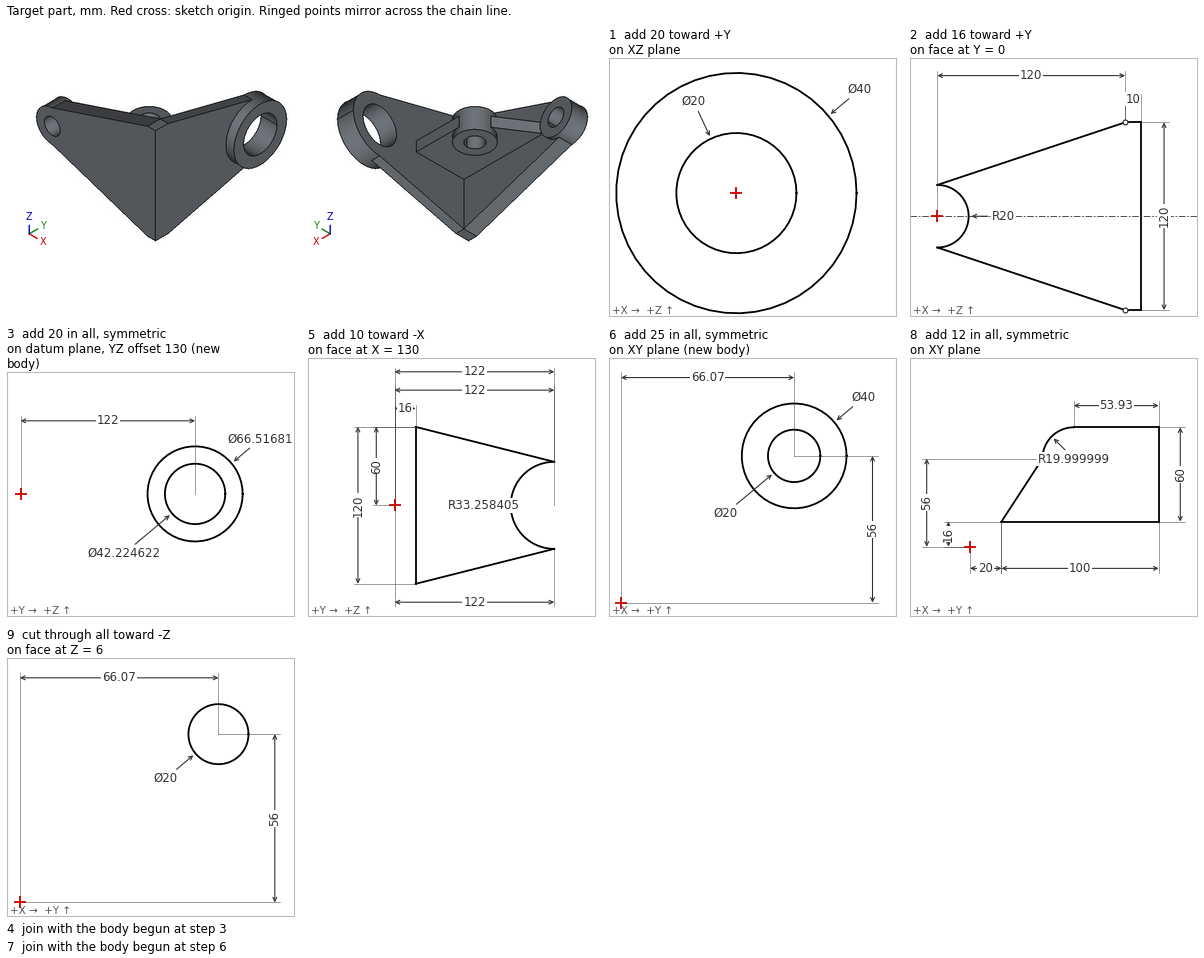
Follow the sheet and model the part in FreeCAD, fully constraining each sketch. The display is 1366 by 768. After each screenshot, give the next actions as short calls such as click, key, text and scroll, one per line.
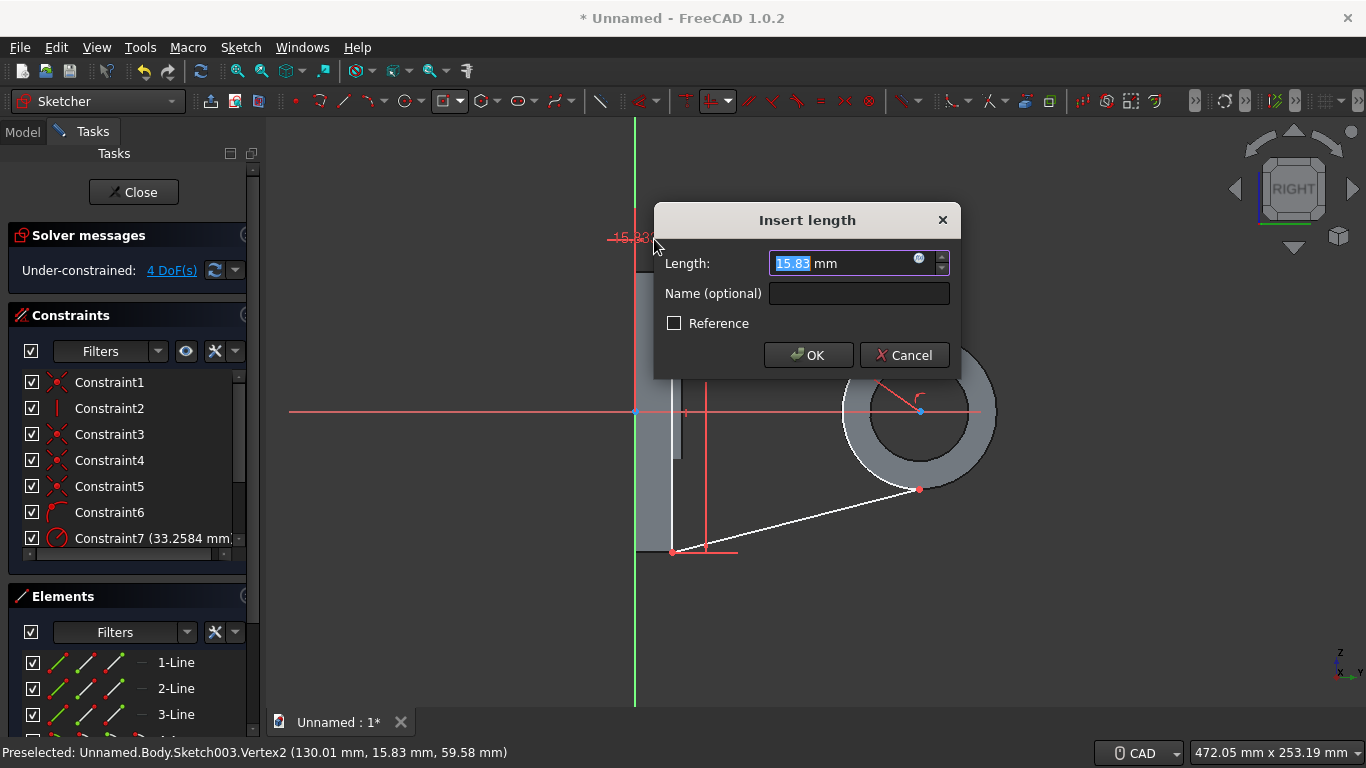
text(16)
key(Return)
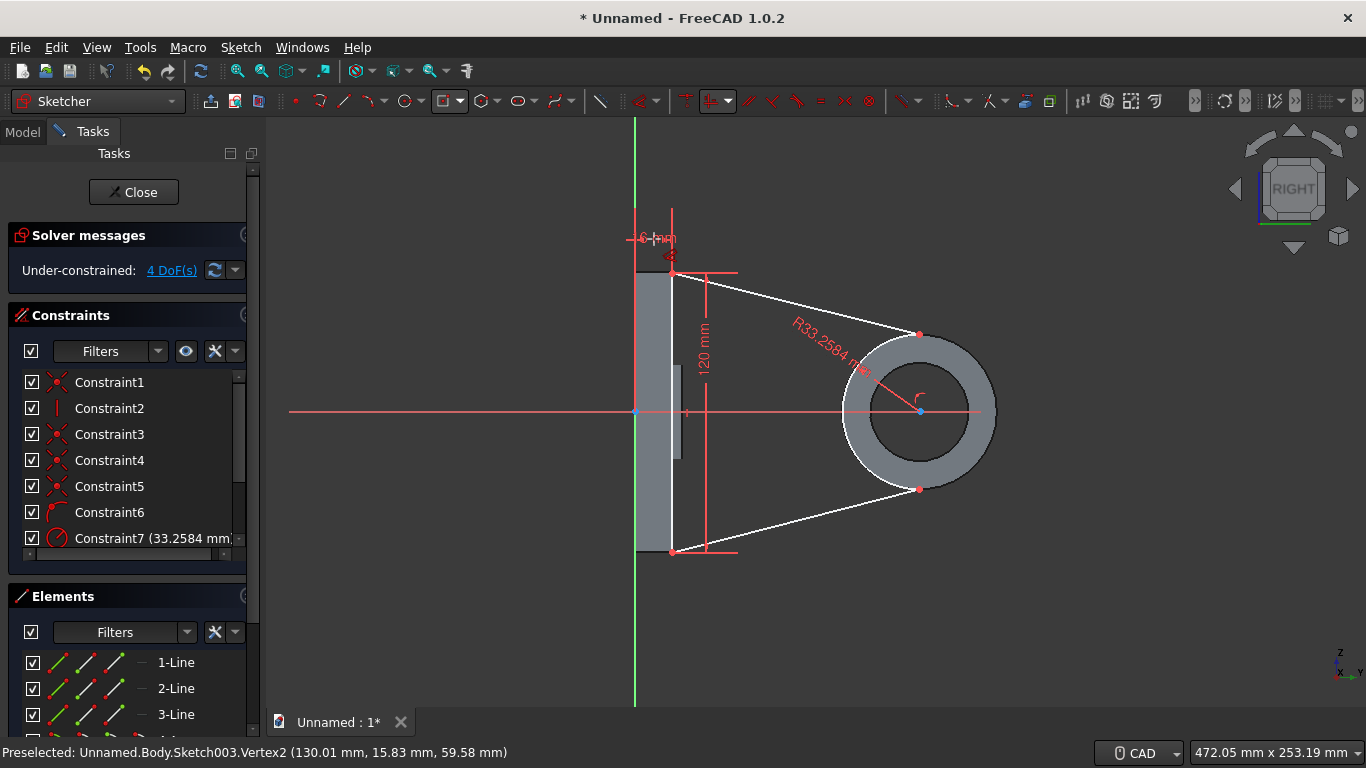
click(672, 273)
click(601, 343)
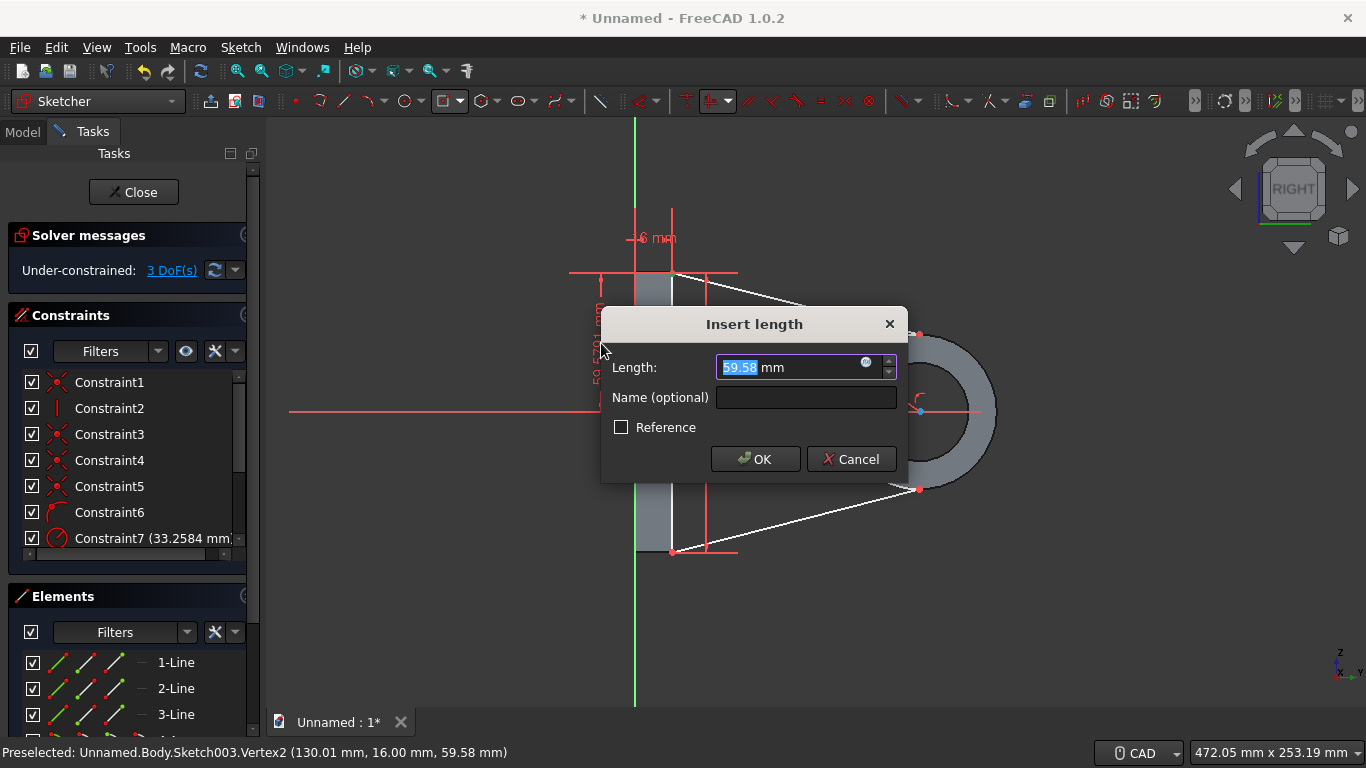
text(60)
key(Return)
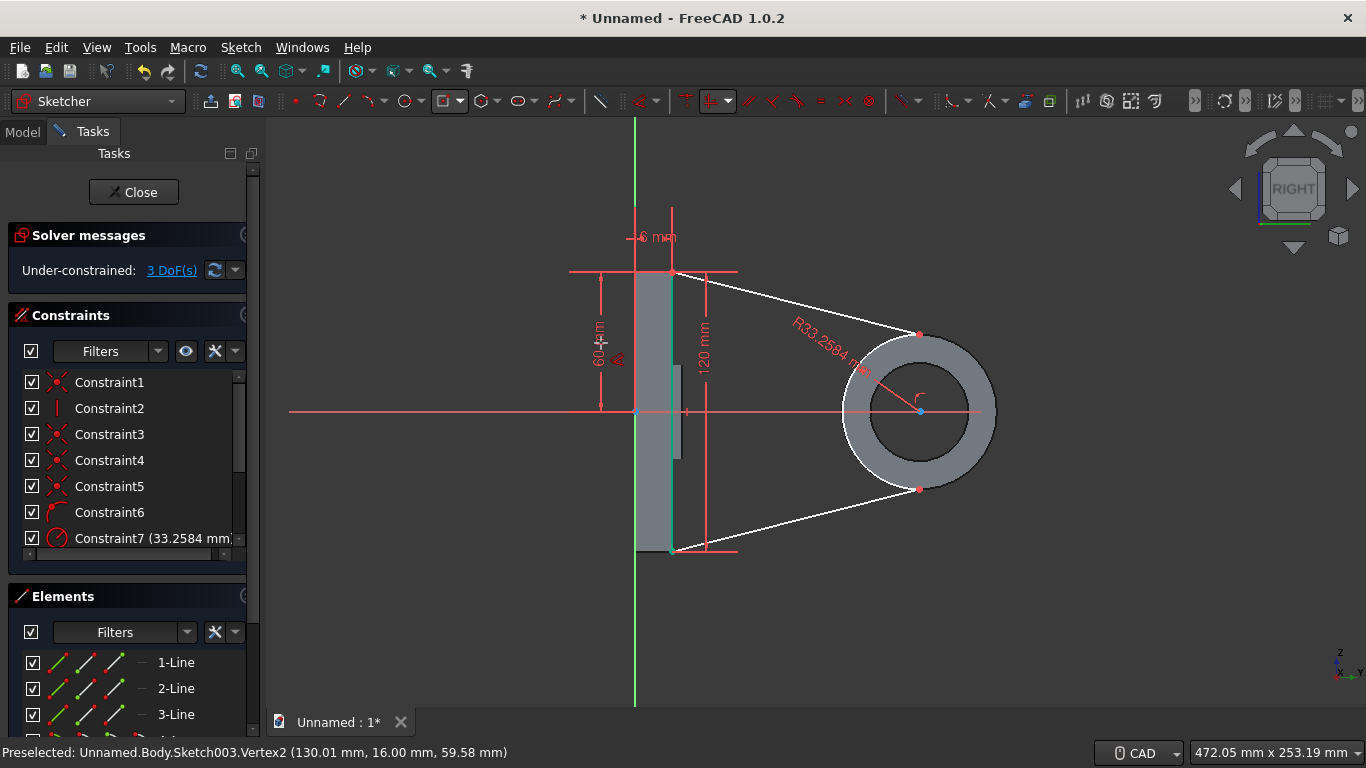
click(919, 335)
click(712, 301)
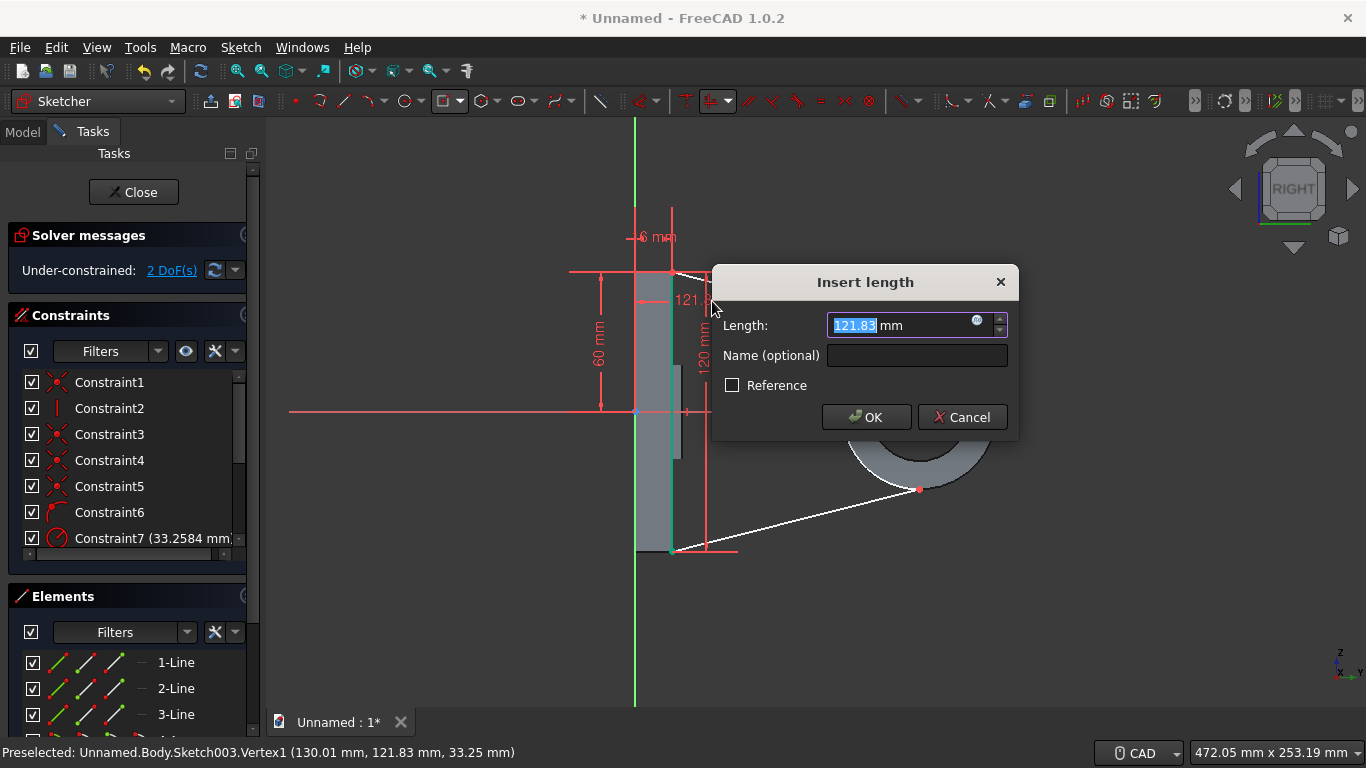
text(122)
key(Return)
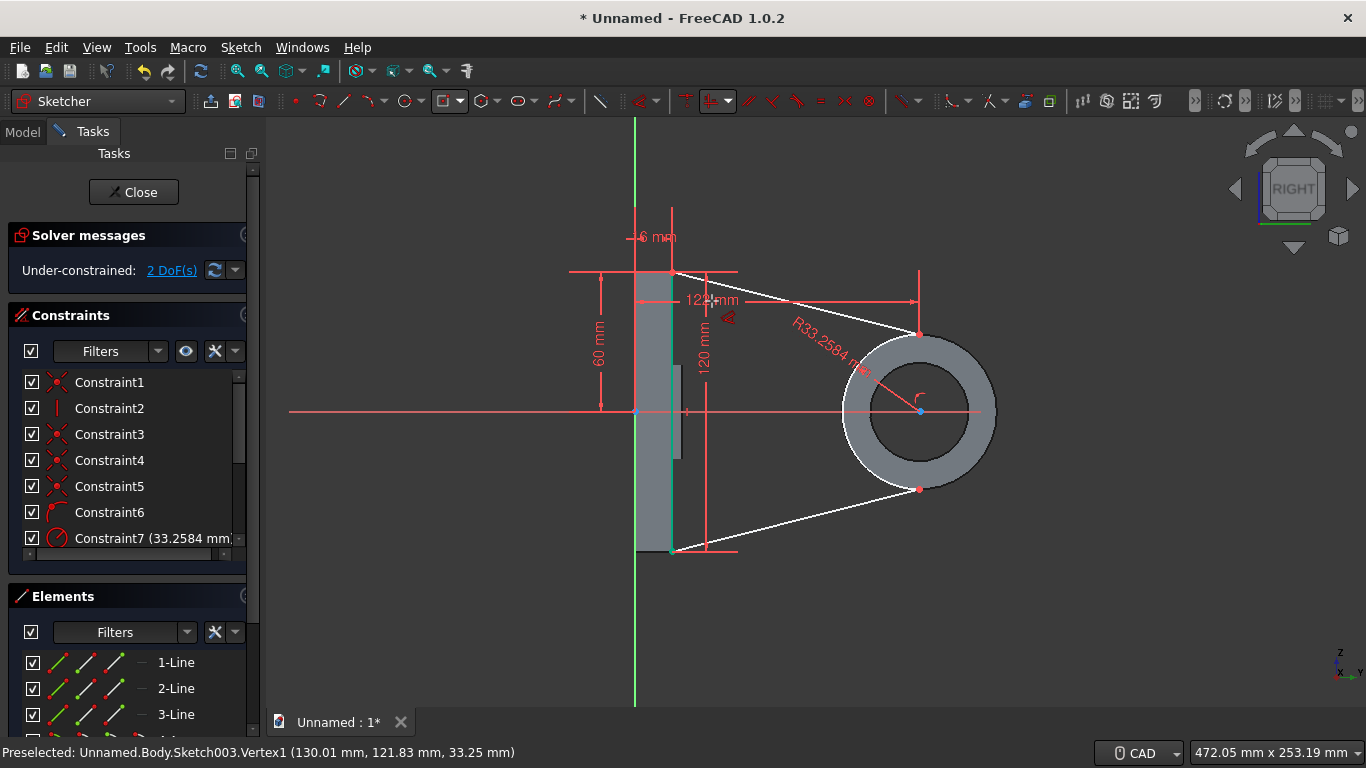
click(919, 489)
click(712, 523)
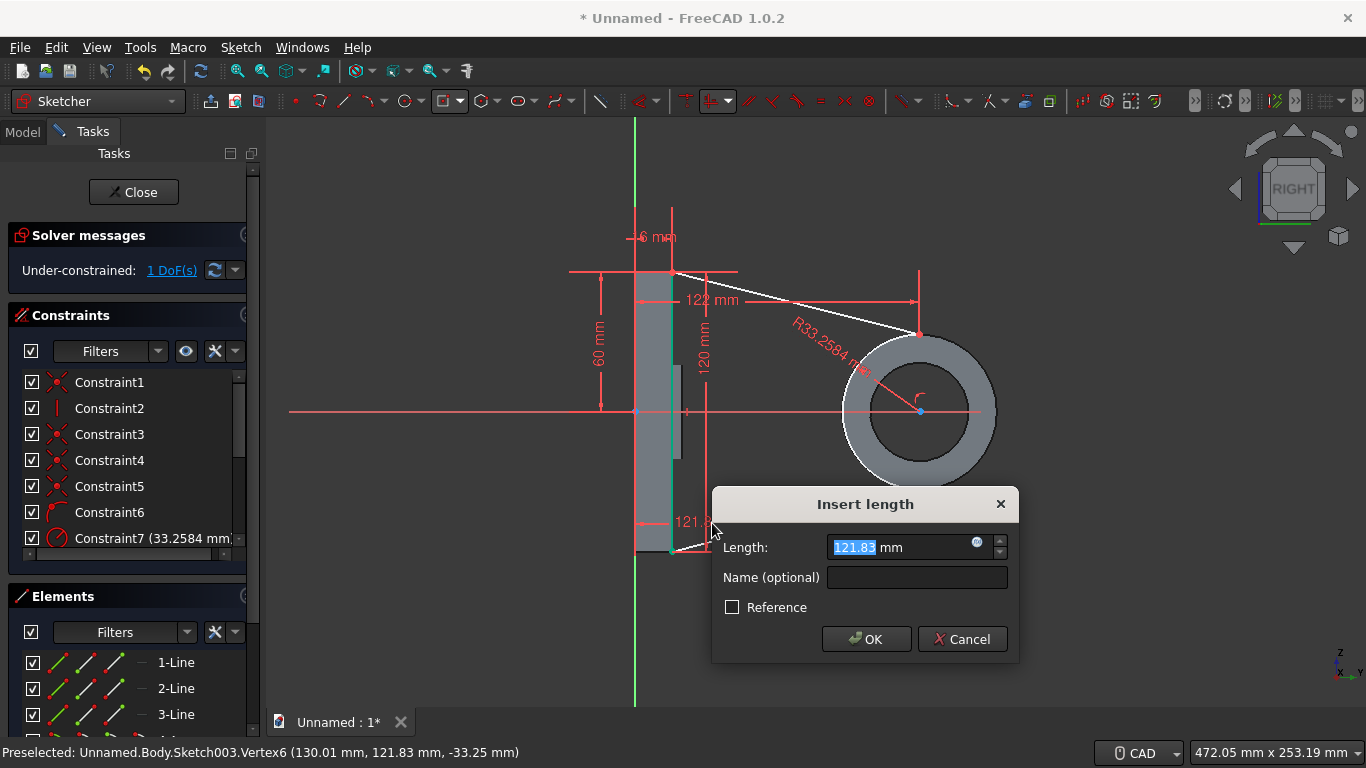
text(122)
key(Return)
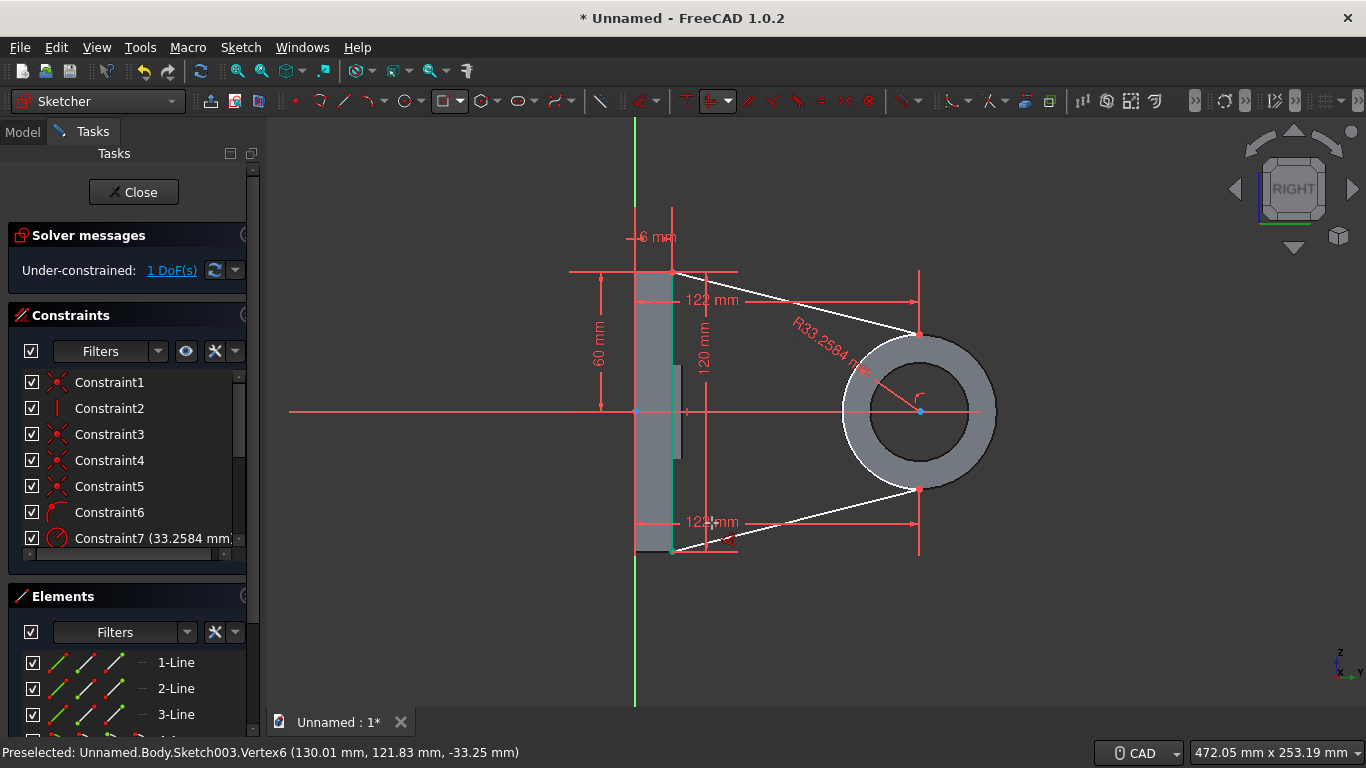
click(920, 412)
click(778, 446)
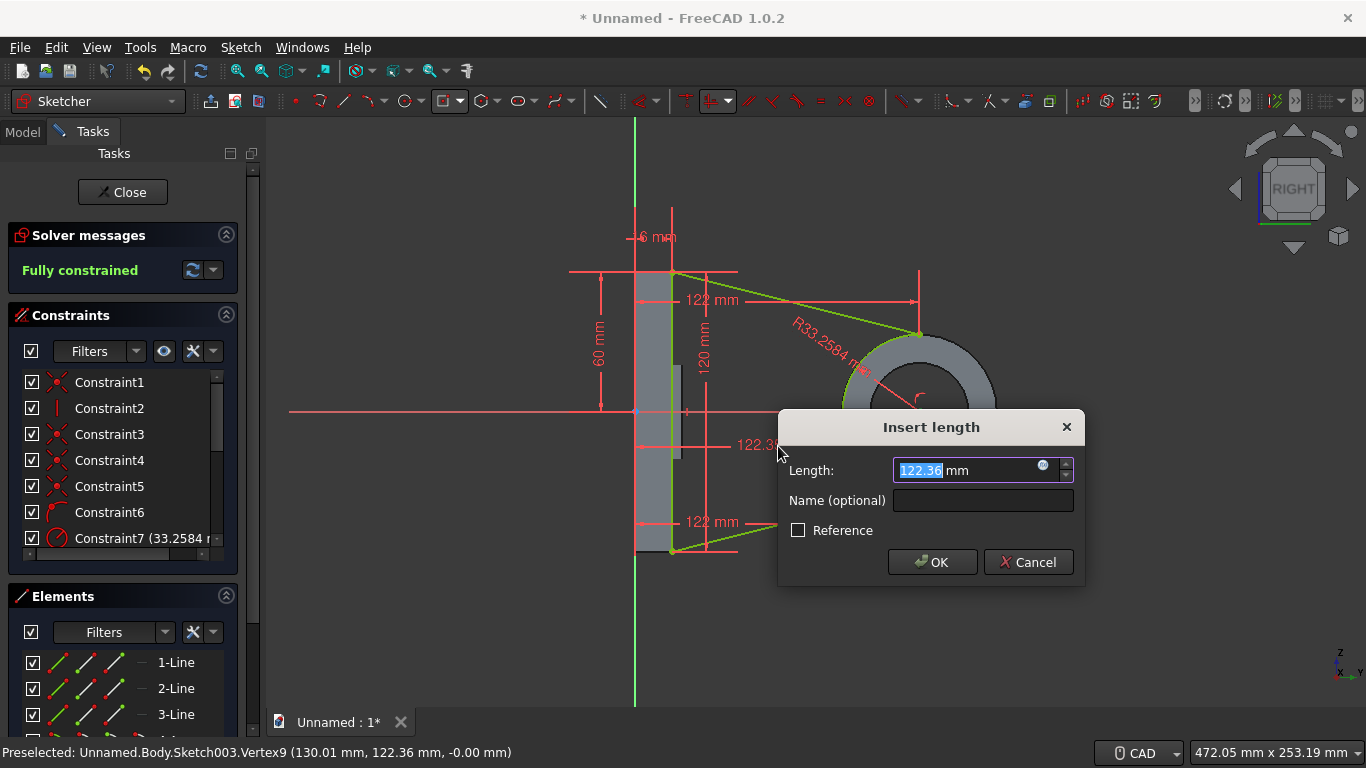
text(122)
key(Return)
key(Escape)